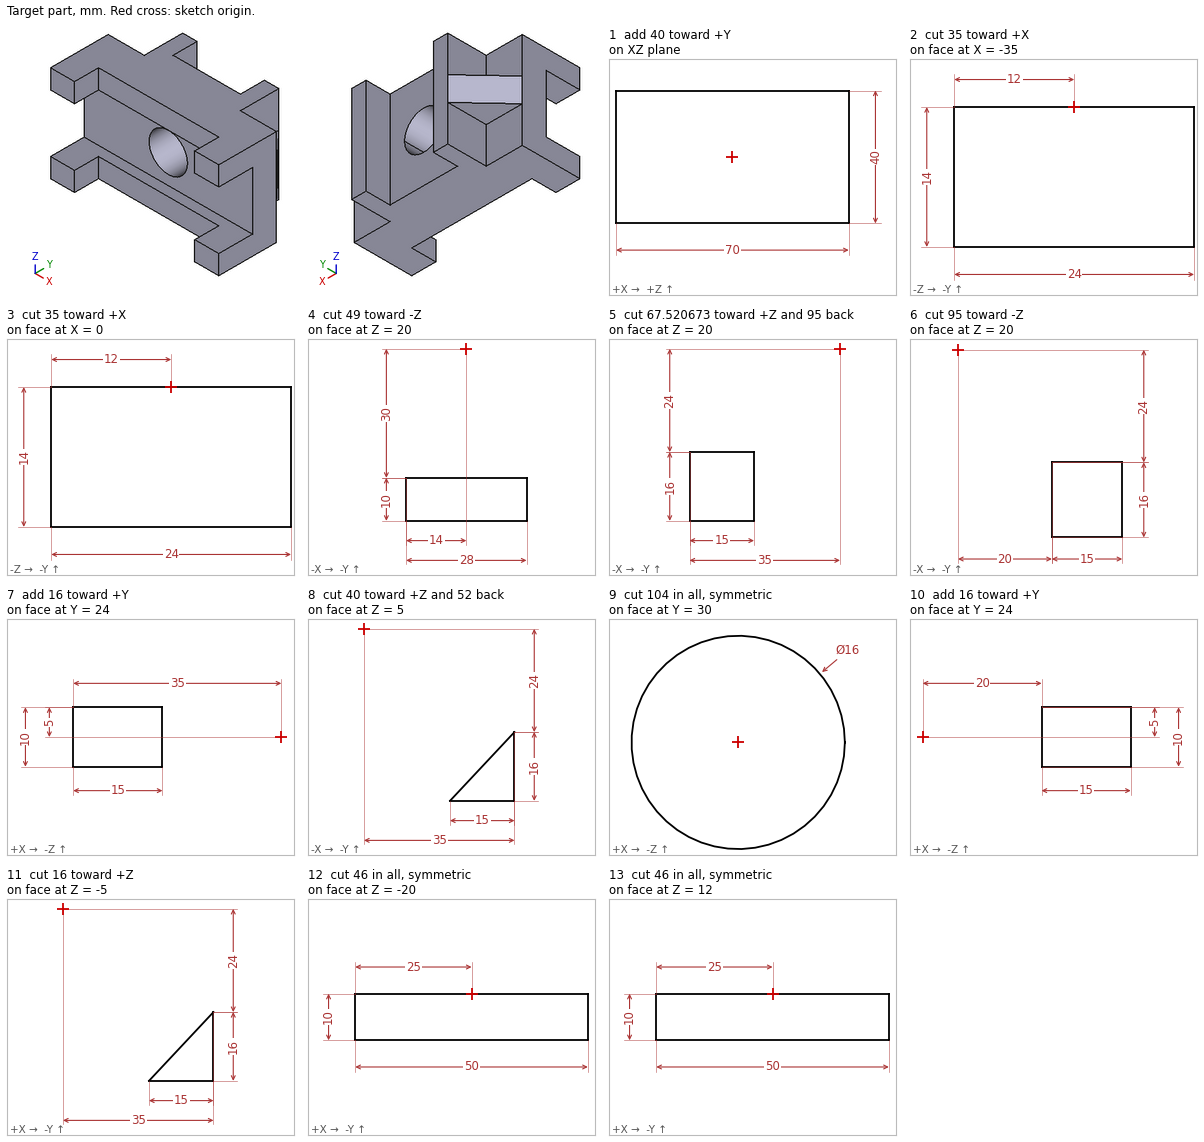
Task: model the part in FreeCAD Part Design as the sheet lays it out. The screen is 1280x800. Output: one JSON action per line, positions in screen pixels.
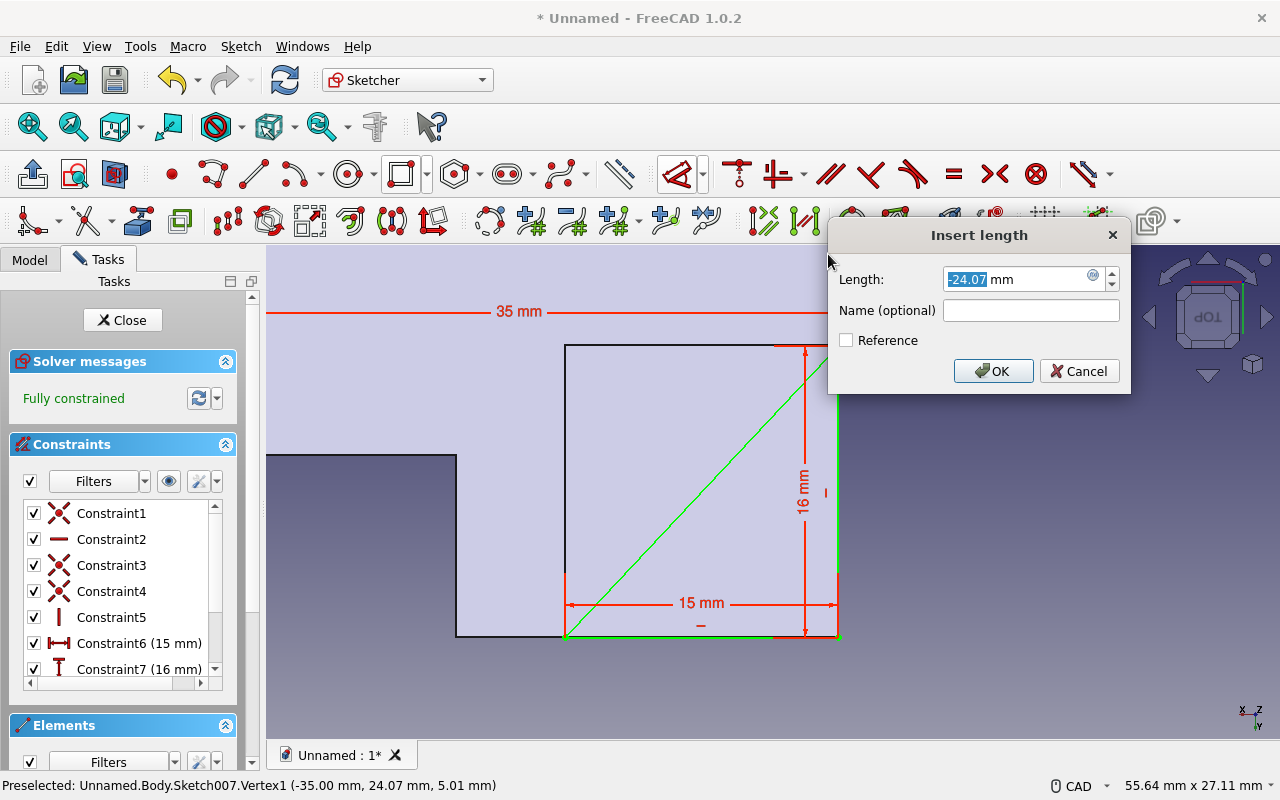
{"action": "type", "text": "-24"}
{"action": "key", "text": "Return"}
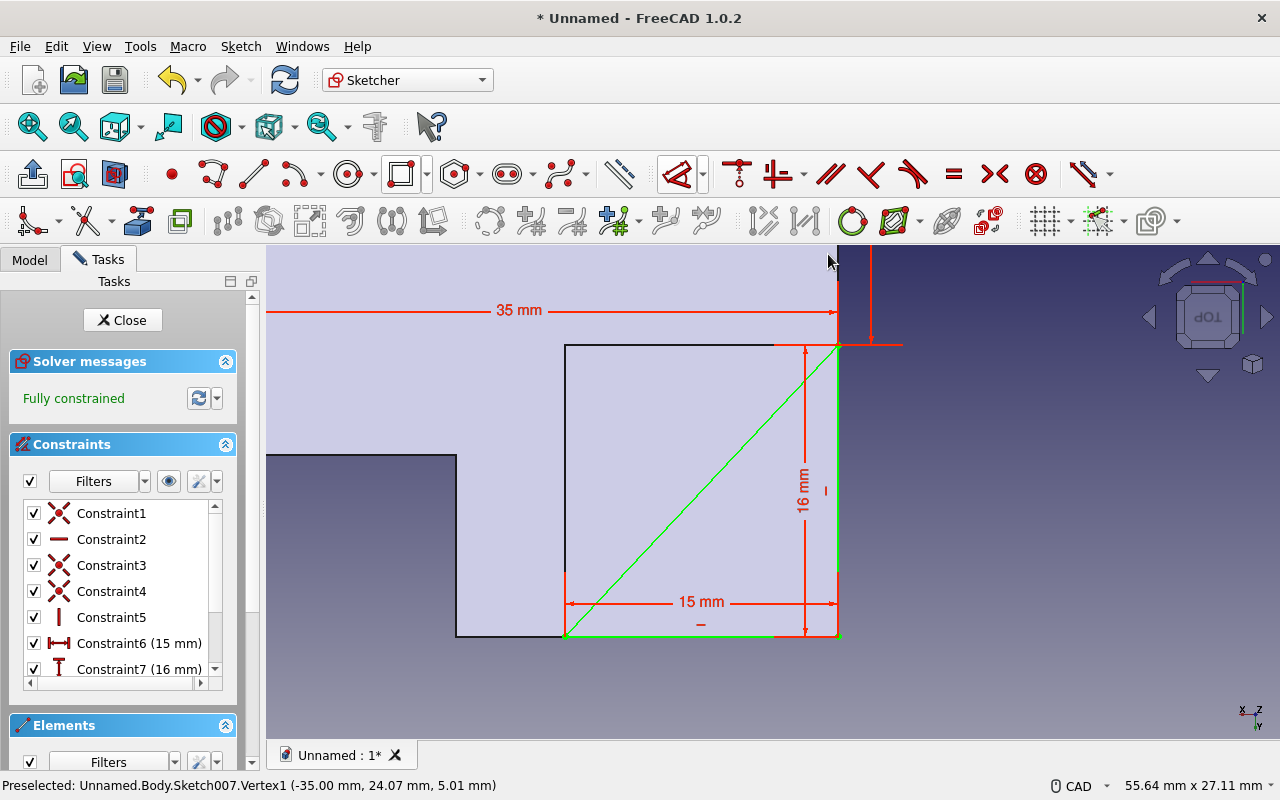
{"action": "left_click", "coordinate": [123, 320]}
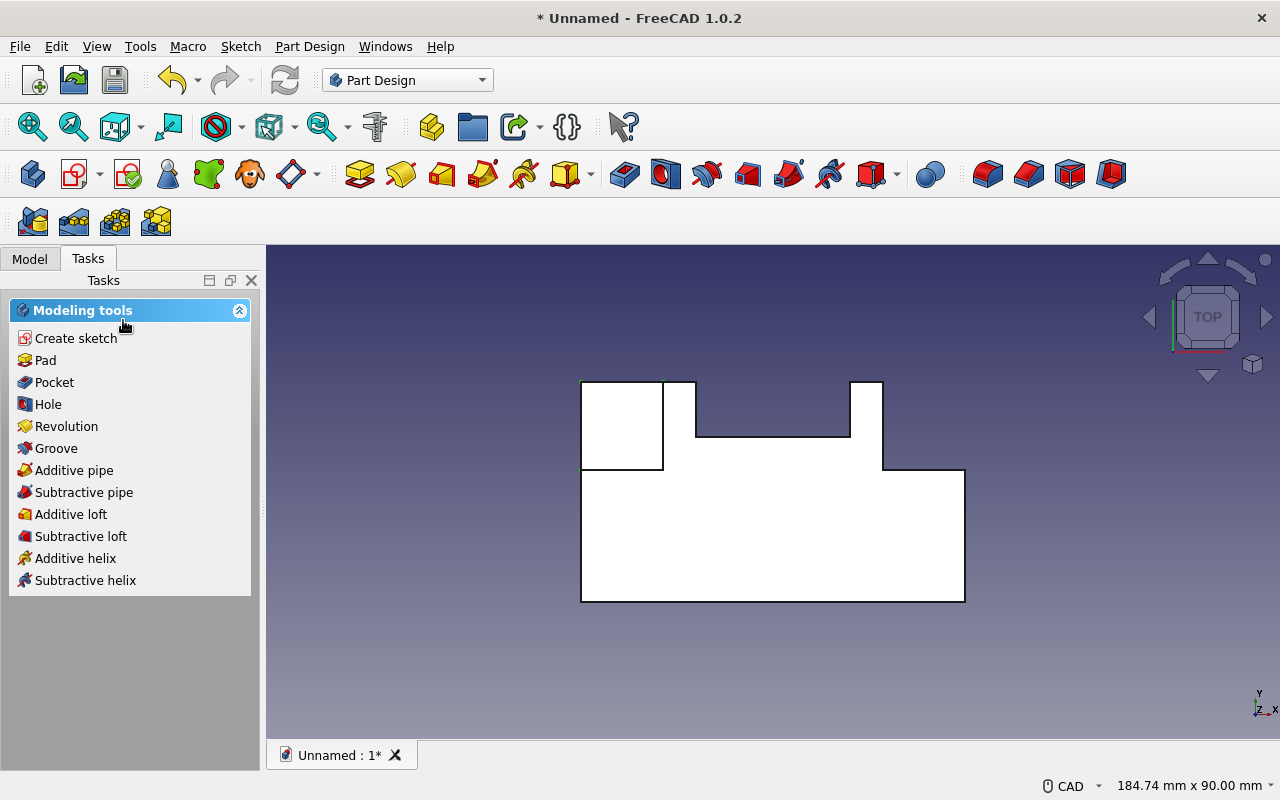
{"action": "left_click", "coordinate": [625, 174]}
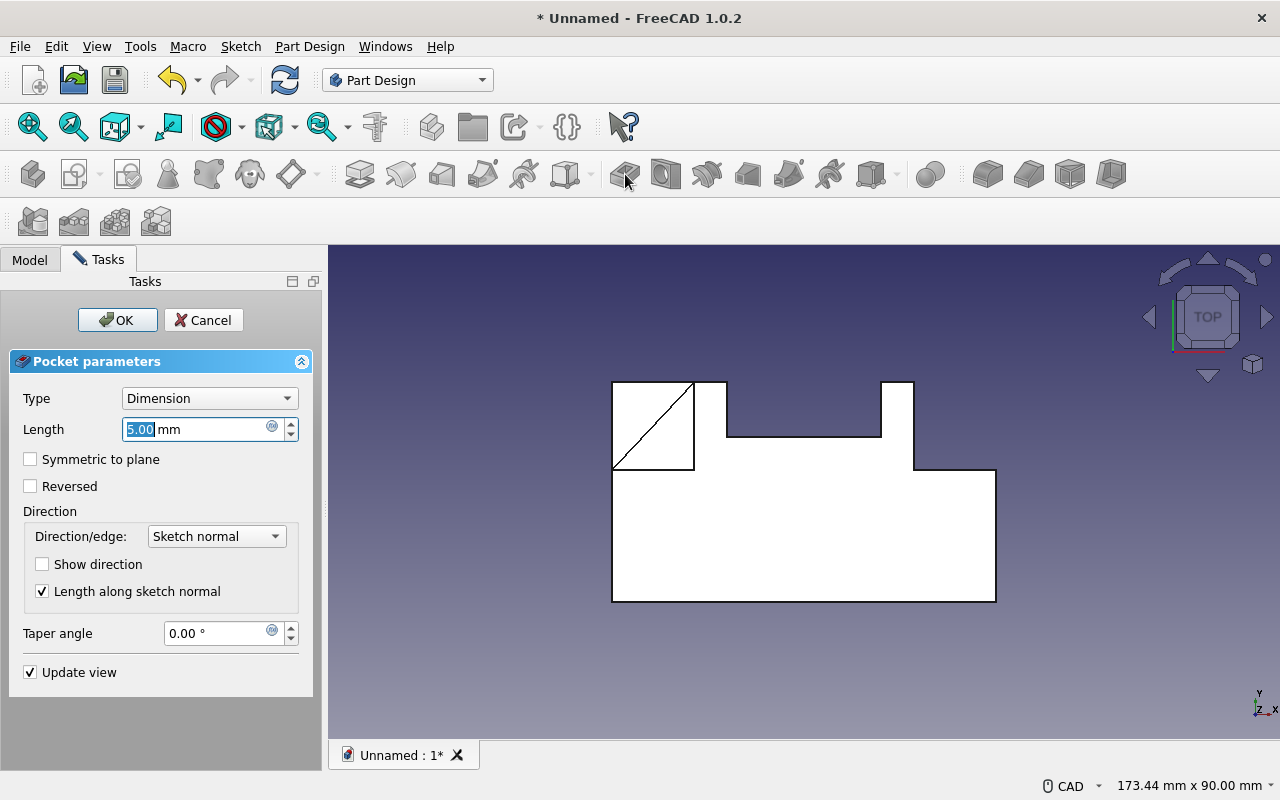
{"action": "left_click", "coordinate": [210, 398]}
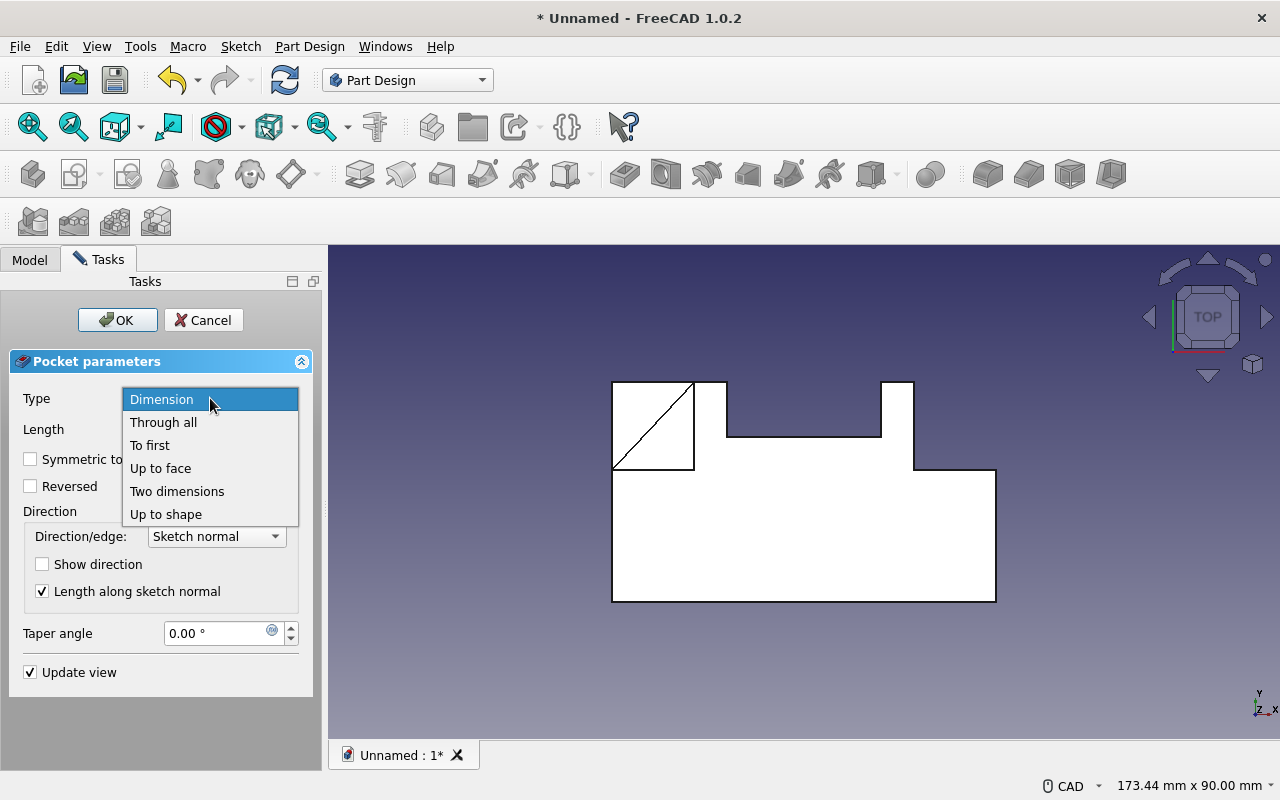
{"action": "left_click", "coordinate": [208, 492]}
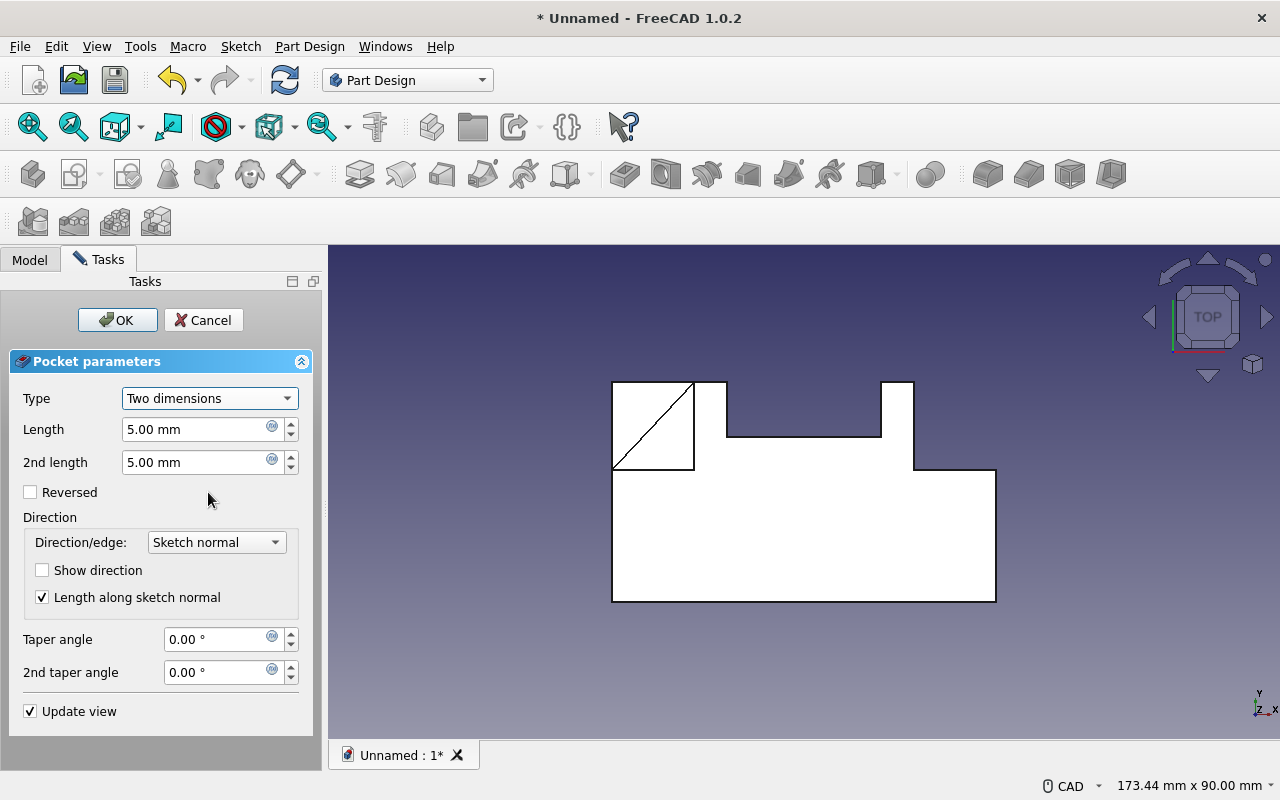
{"action": "triple_click", "coordinate": [204, 430]}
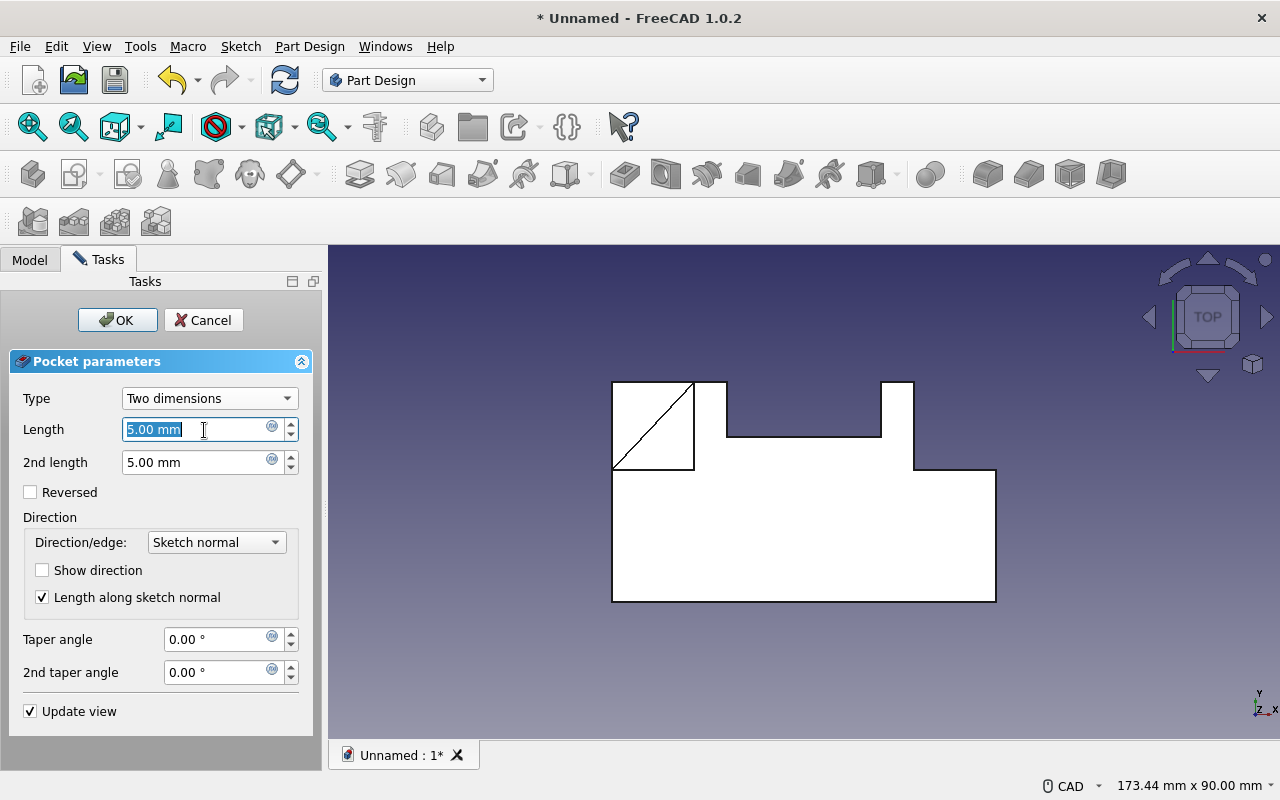
{"action": "type", "text": "40"}
{"action": "key", "text": "Tab"}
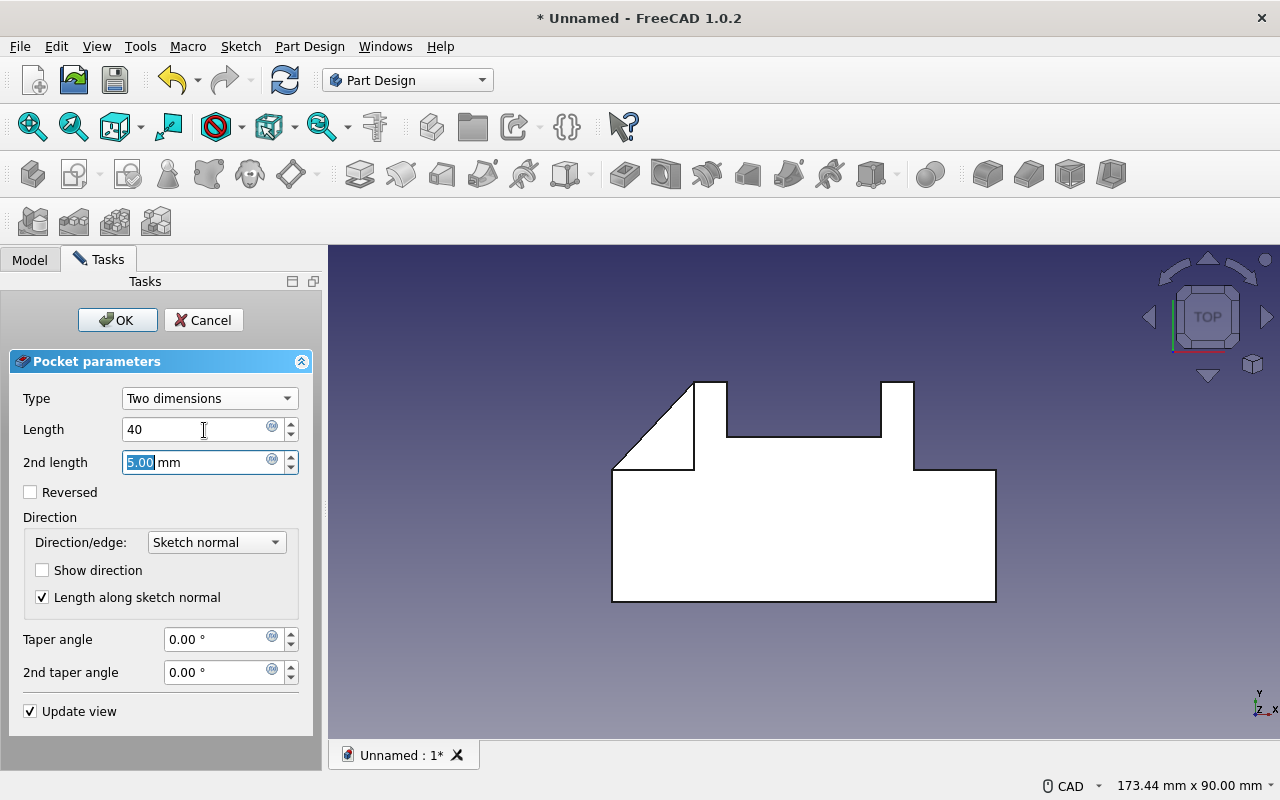
{"action": "type", "text": "52"}
{"action": "key", "text": "Tab"}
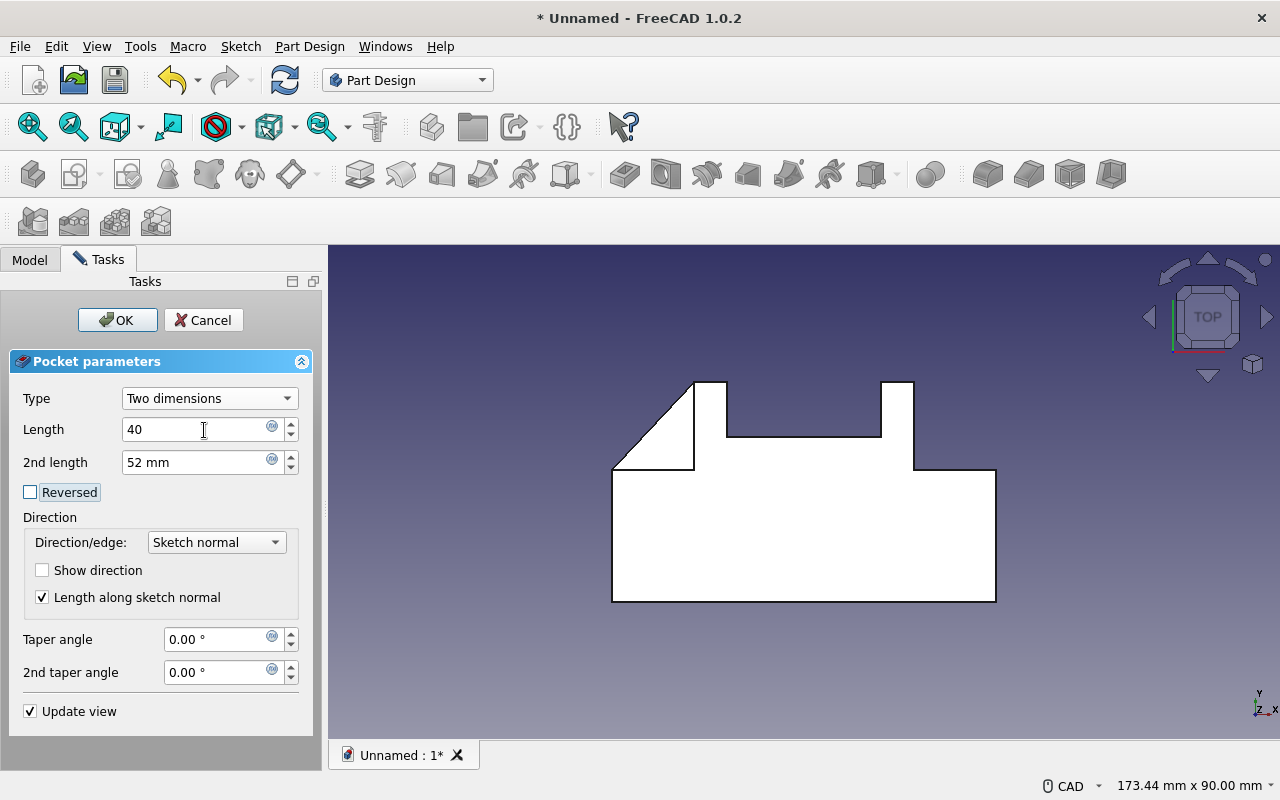
{"action": "left_click", "coordinate": [31, 492]}